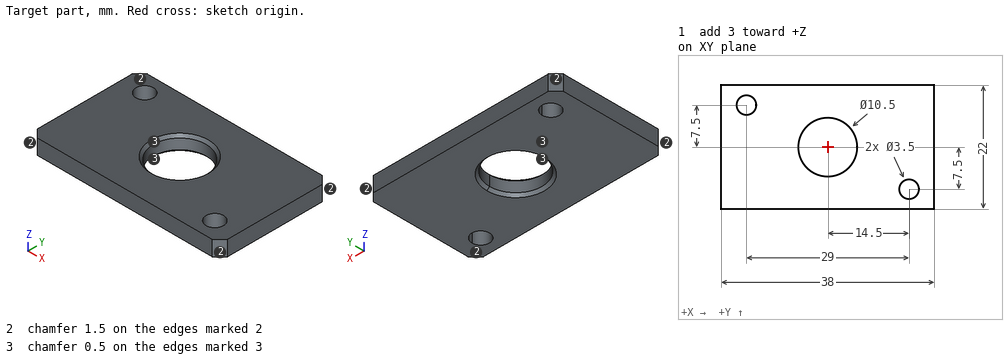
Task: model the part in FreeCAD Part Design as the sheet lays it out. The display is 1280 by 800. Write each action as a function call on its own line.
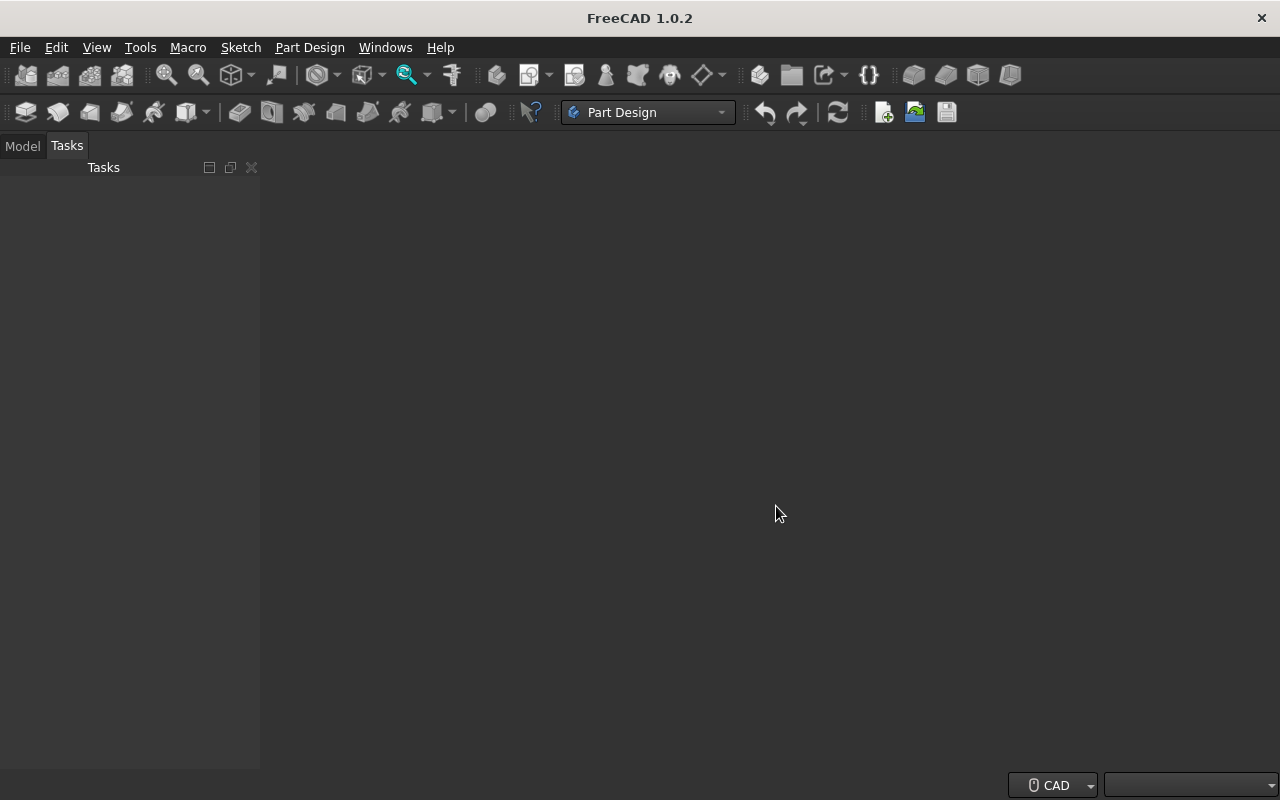
click(884, 112)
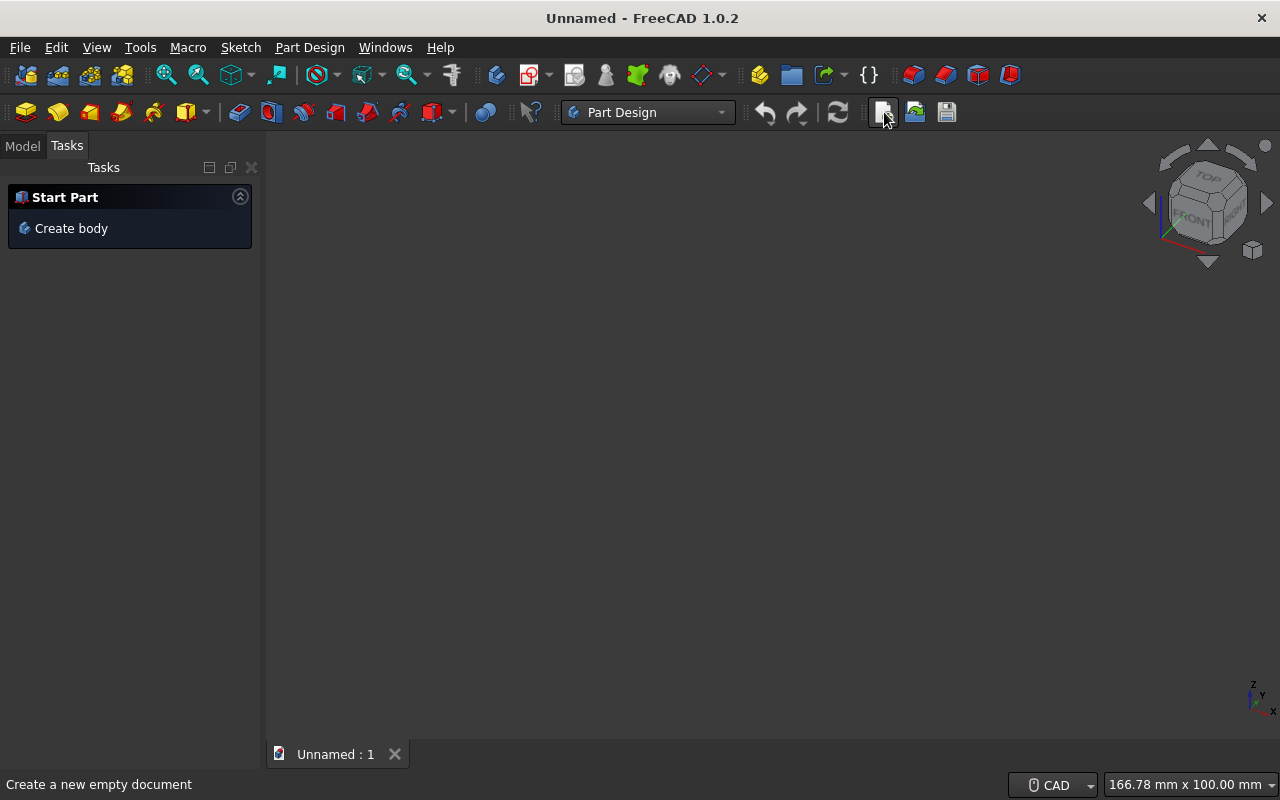
click(530, 76)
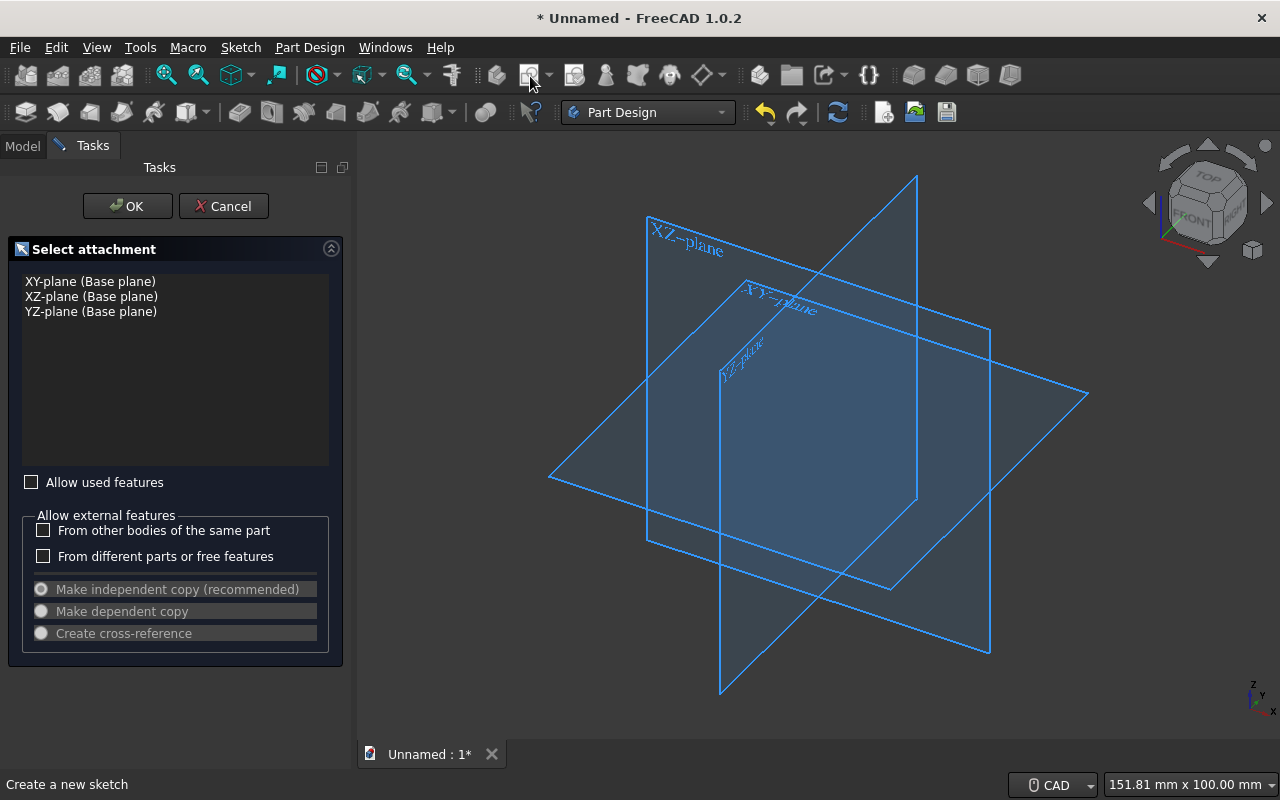
click(82, 282)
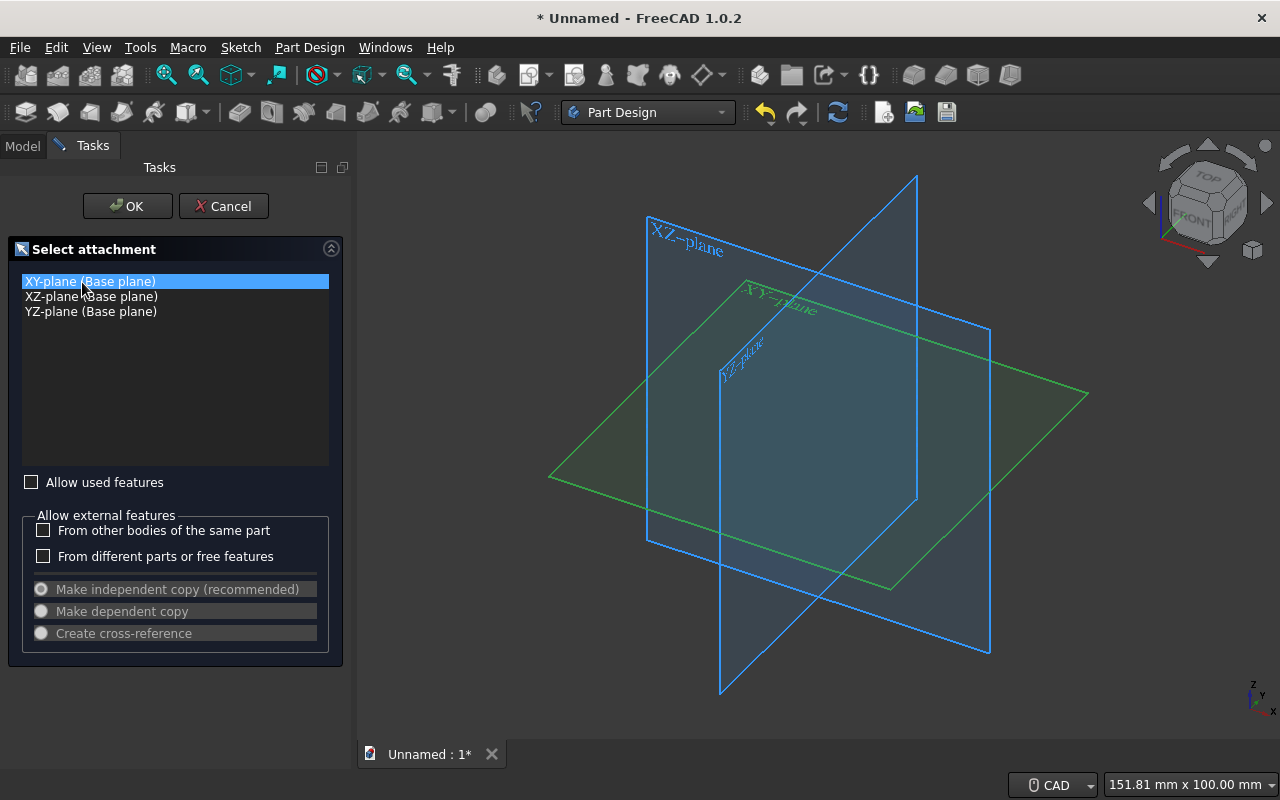
click(128, 206)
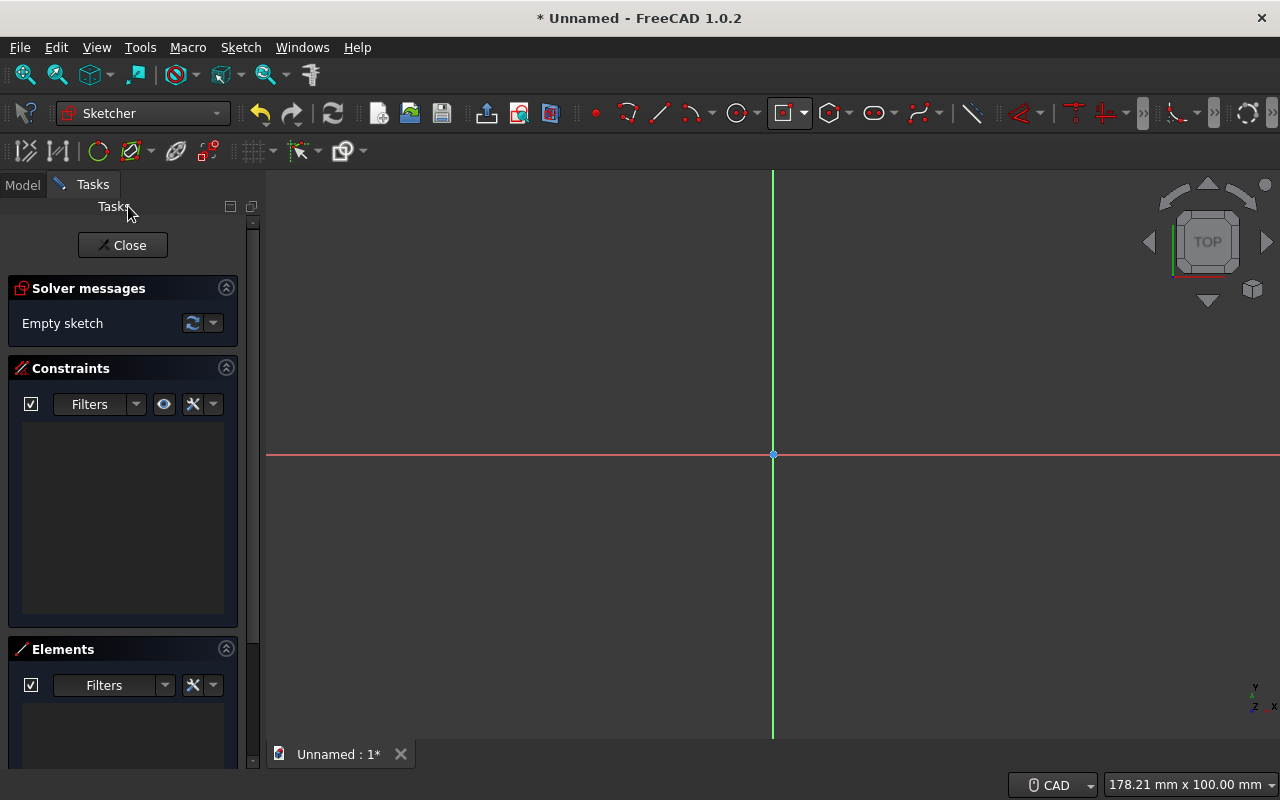
scroll(813, 454, up, 5)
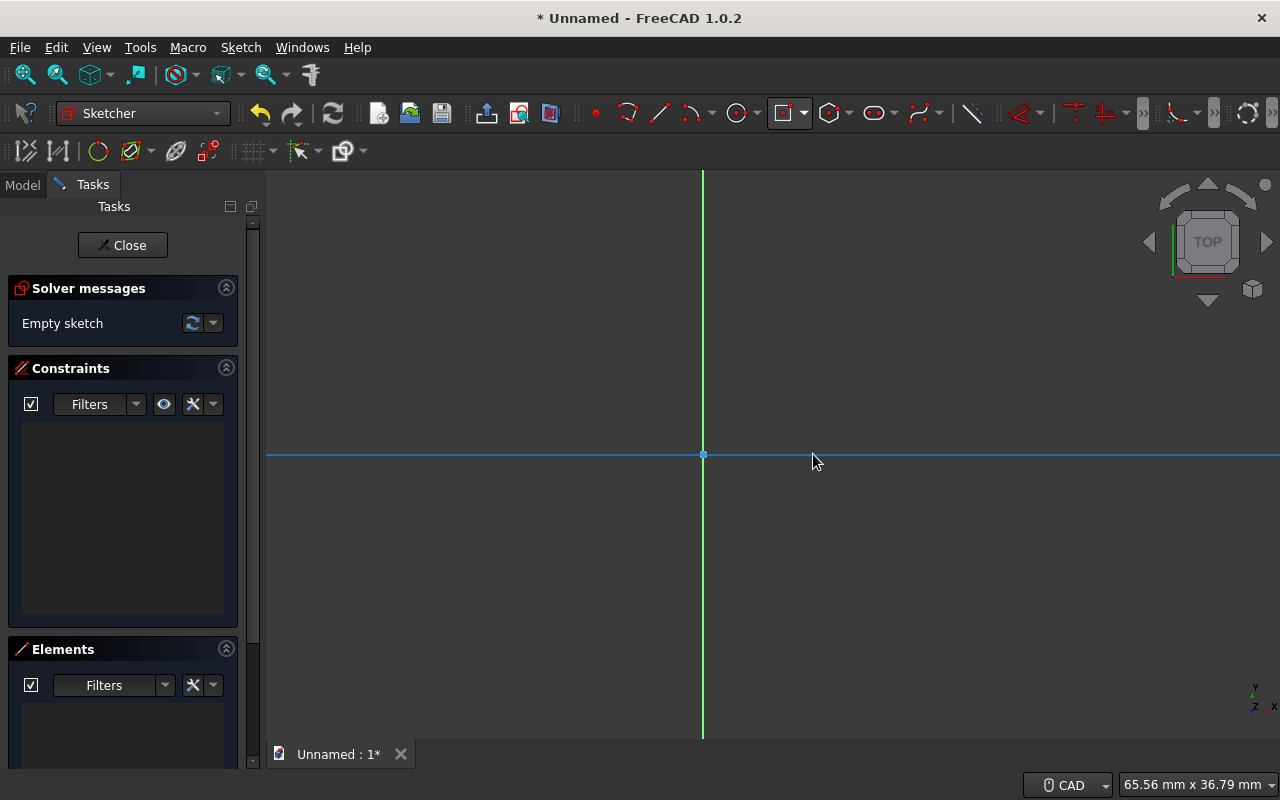
click(784, 114)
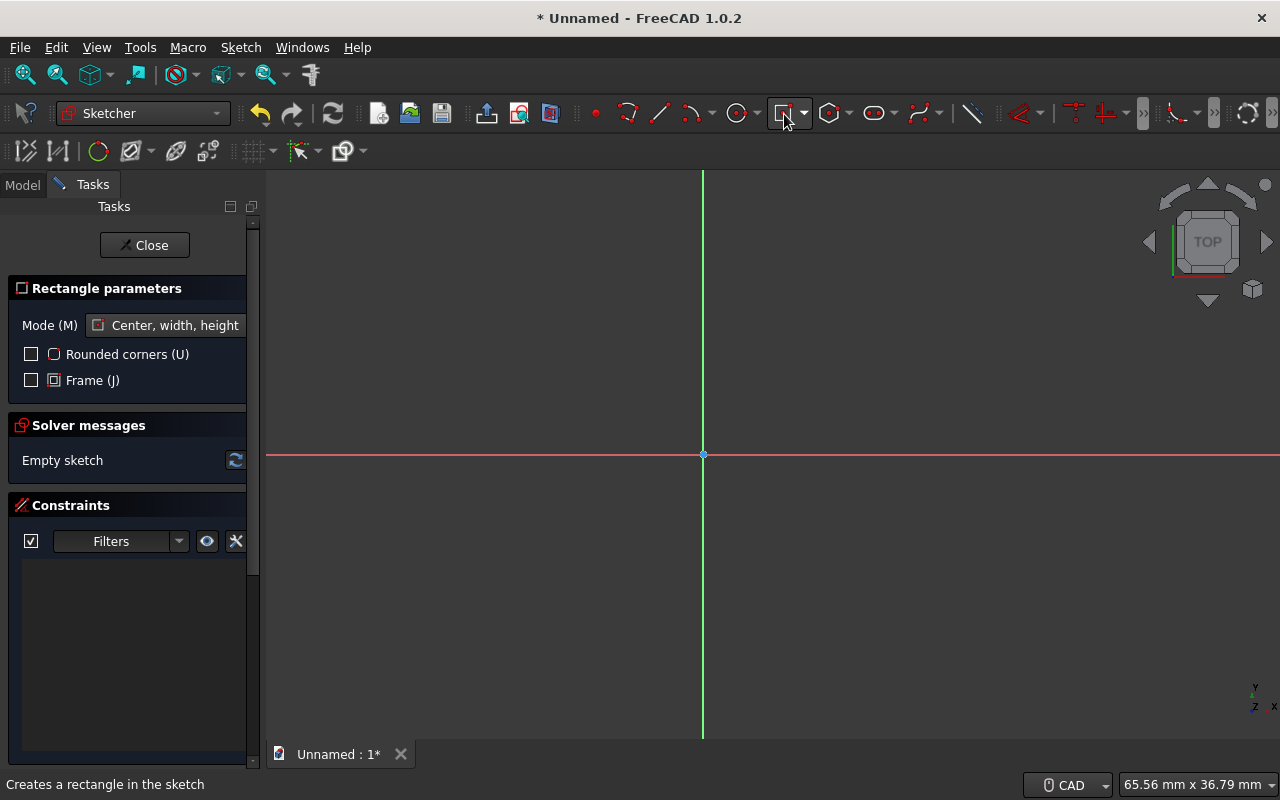
click(703, 454)
move(997, 284)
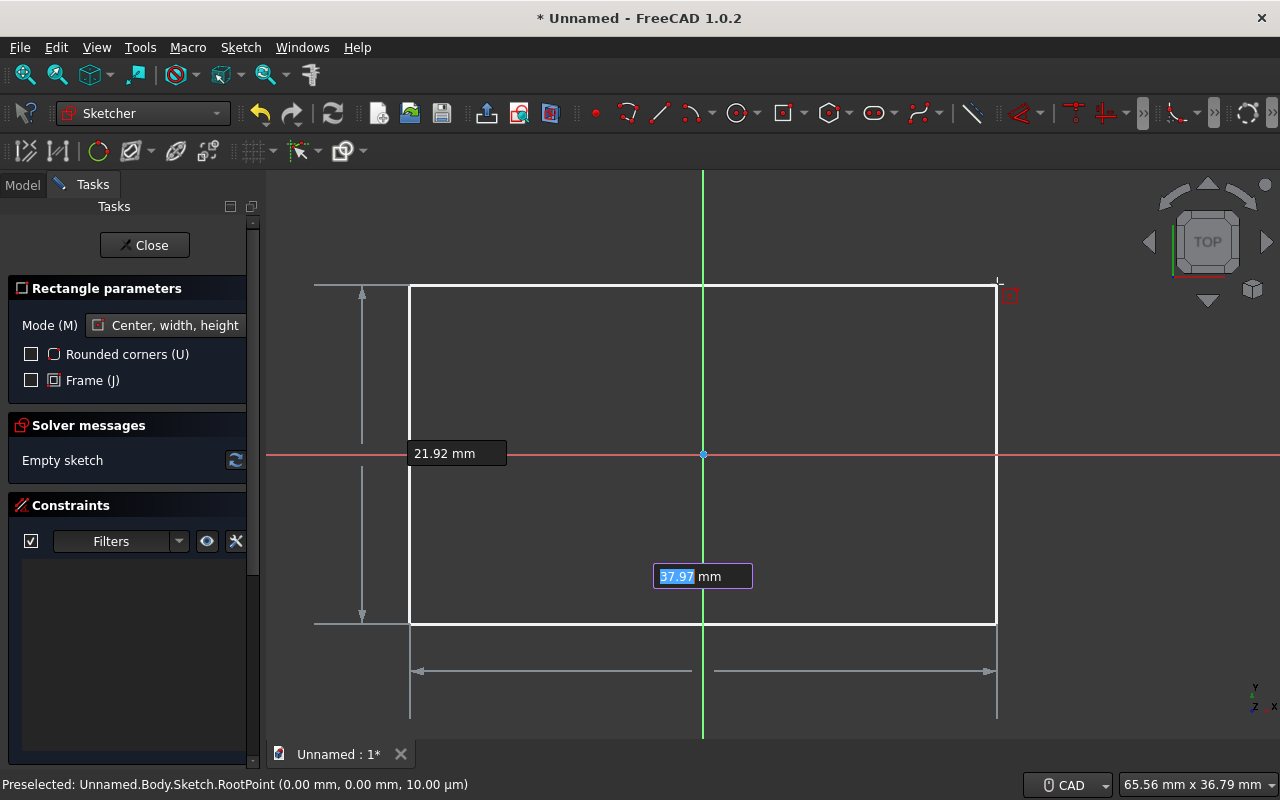
text(38)
key(Tab)
text(22)
key(Return)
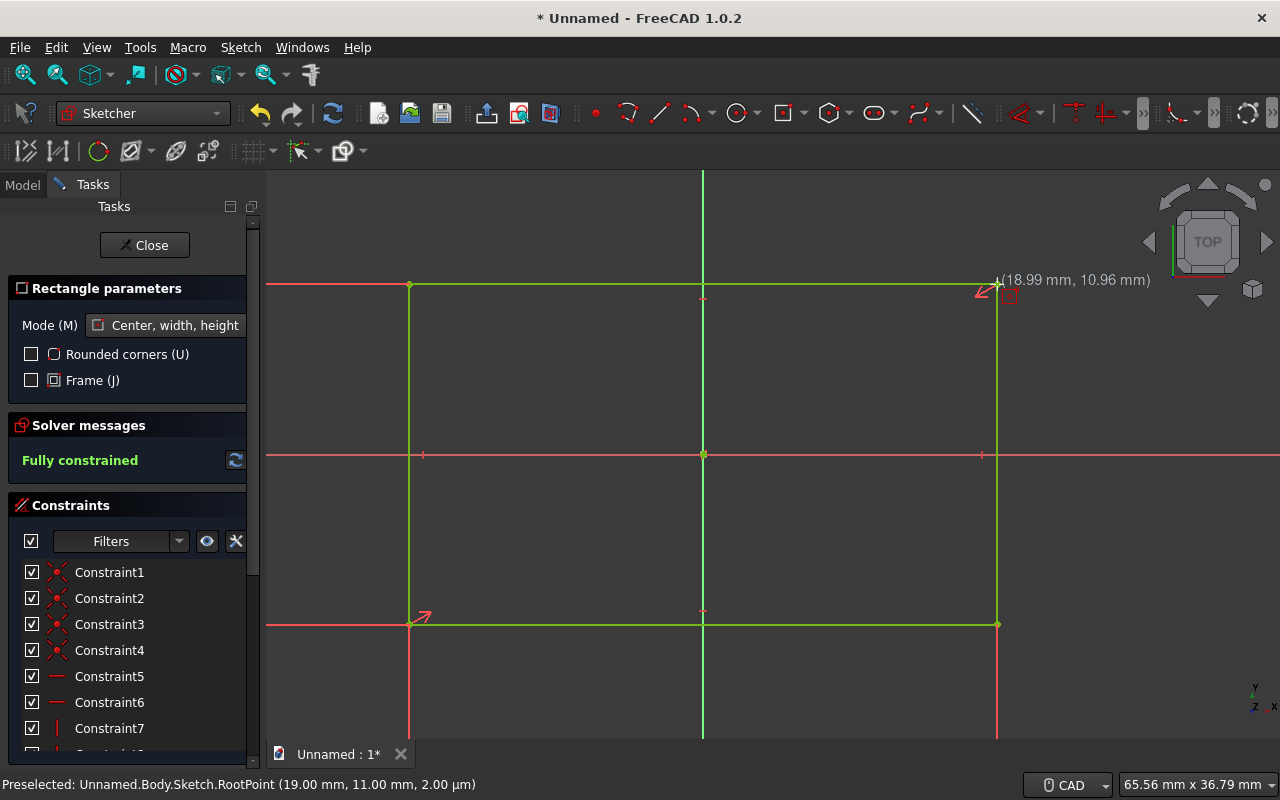
key(g)
key(c)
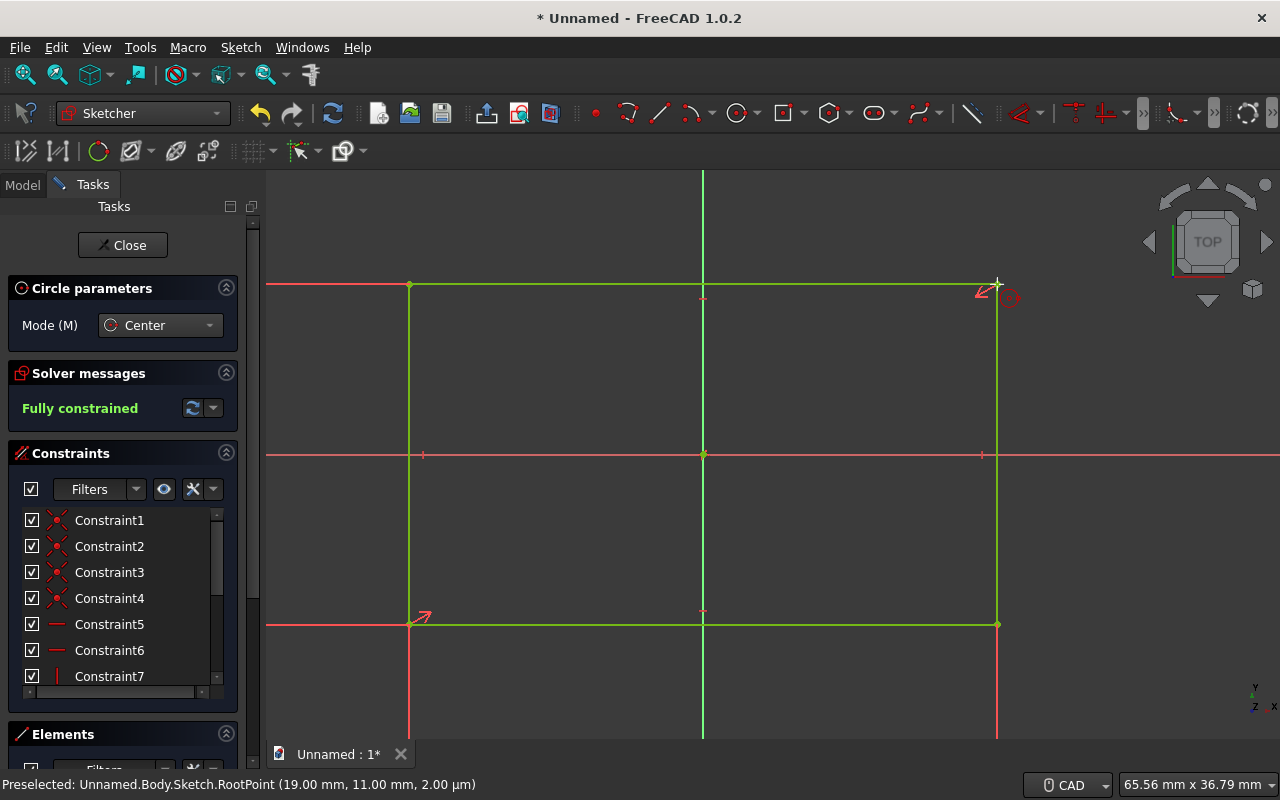
click(928, 571)
move(947, 551)